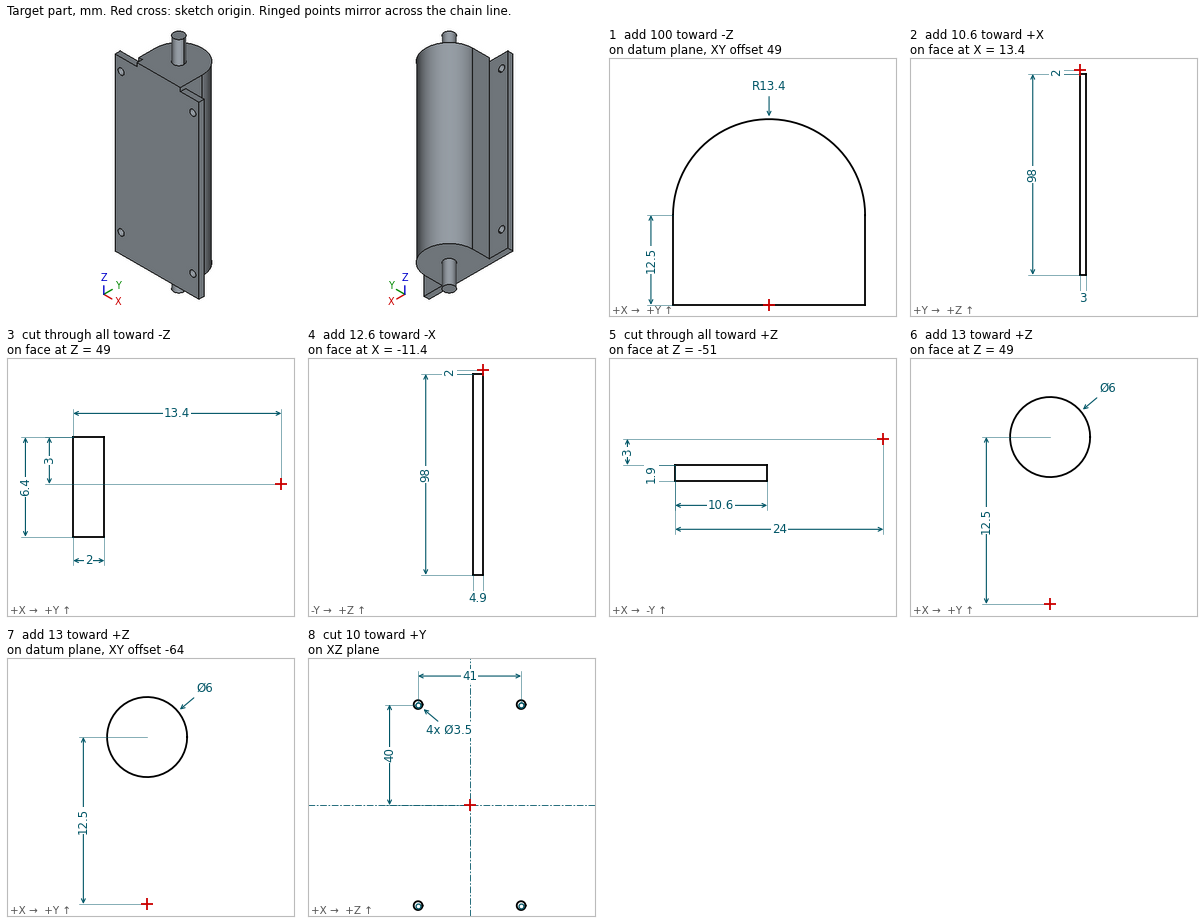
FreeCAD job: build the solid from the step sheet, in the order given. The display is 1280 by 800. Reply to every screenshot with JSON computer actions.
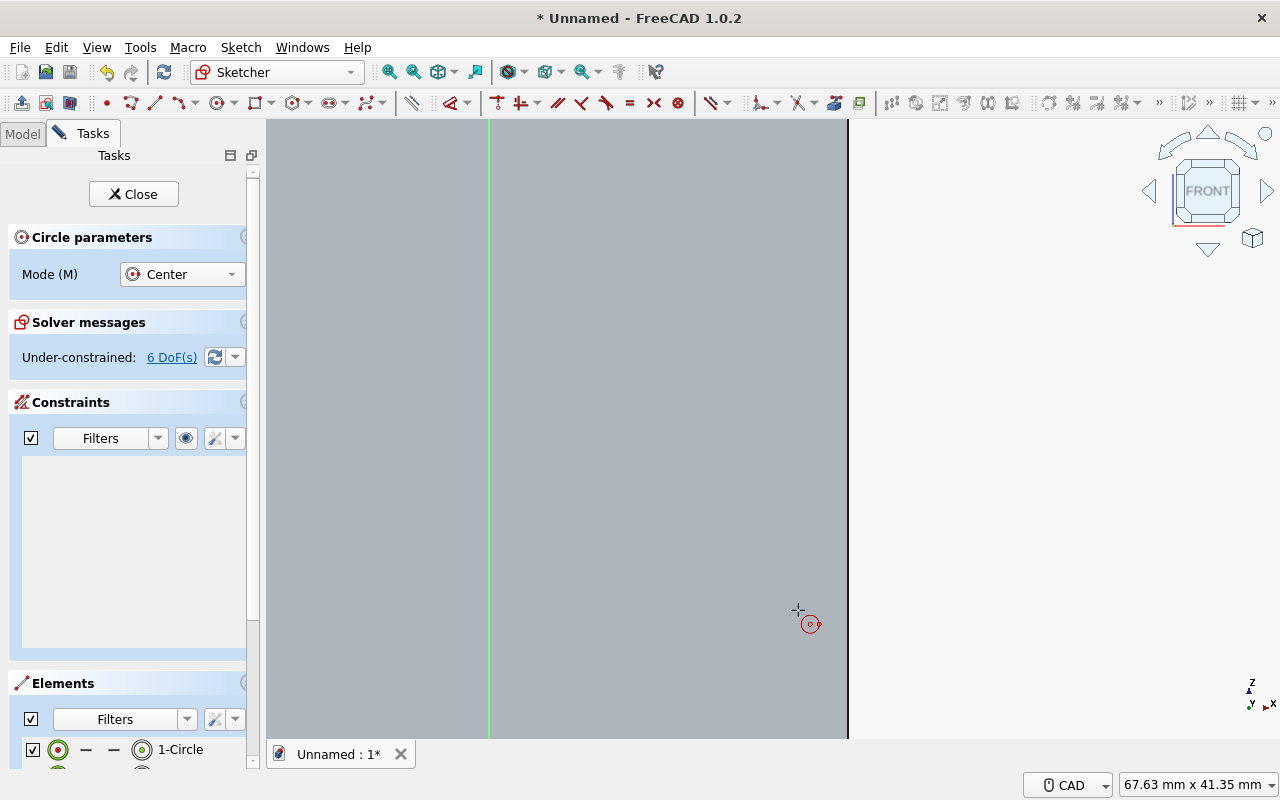
{"action": "left_click", "coordinate": [796, 608]}
{"action": "left_click", "coordinate": [814, 590]}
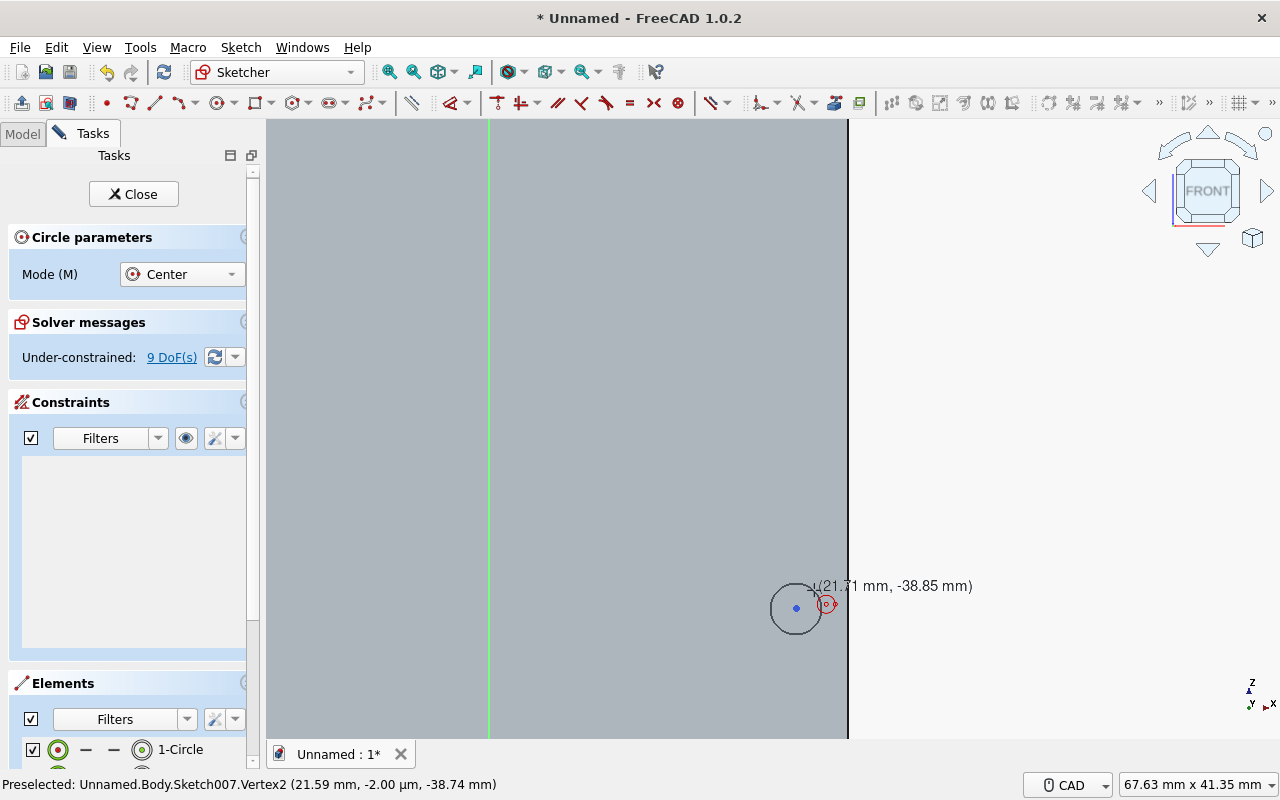
{"action": "scroll", "coordinate": [798, 610], "scroll_direction": "down", "scroll_amount": 6}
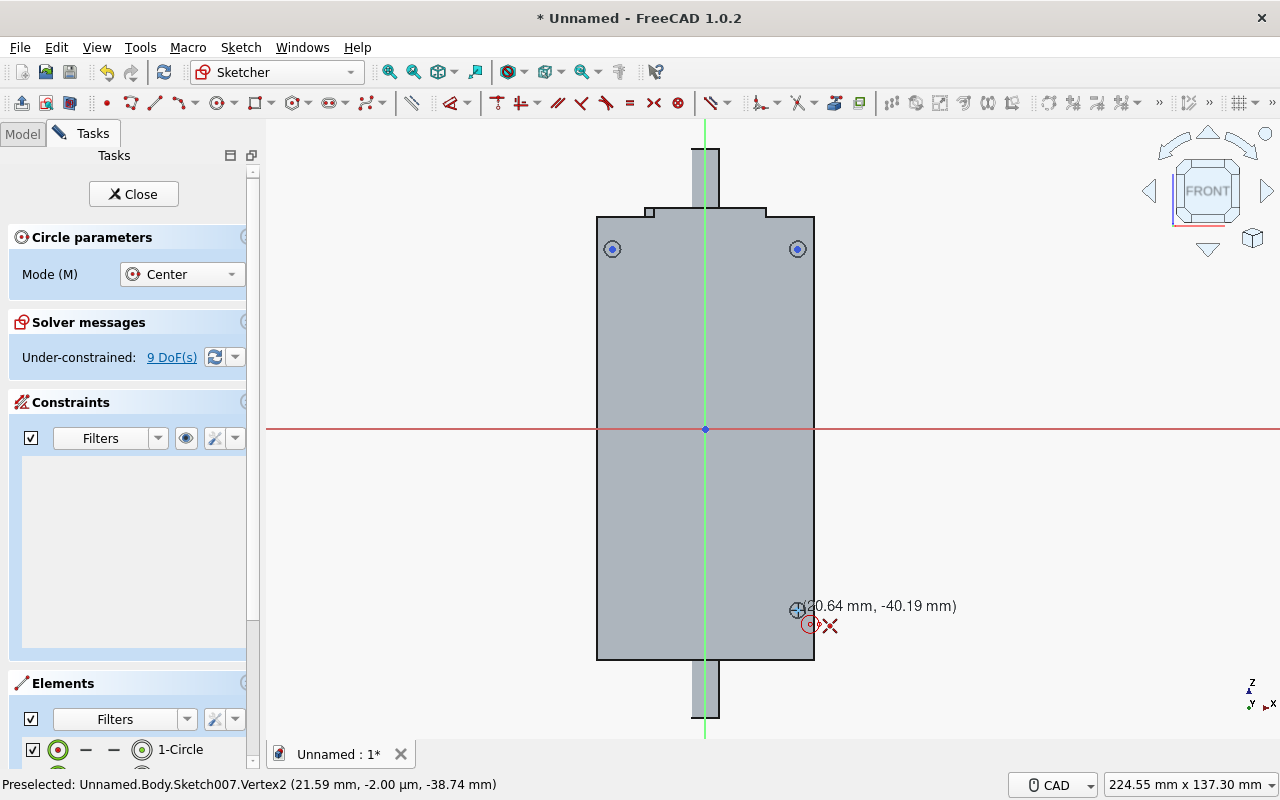
{"action": "scroll", "coordinate": [613, 610], "scroll_direction": "up", "scroll_amount": 6}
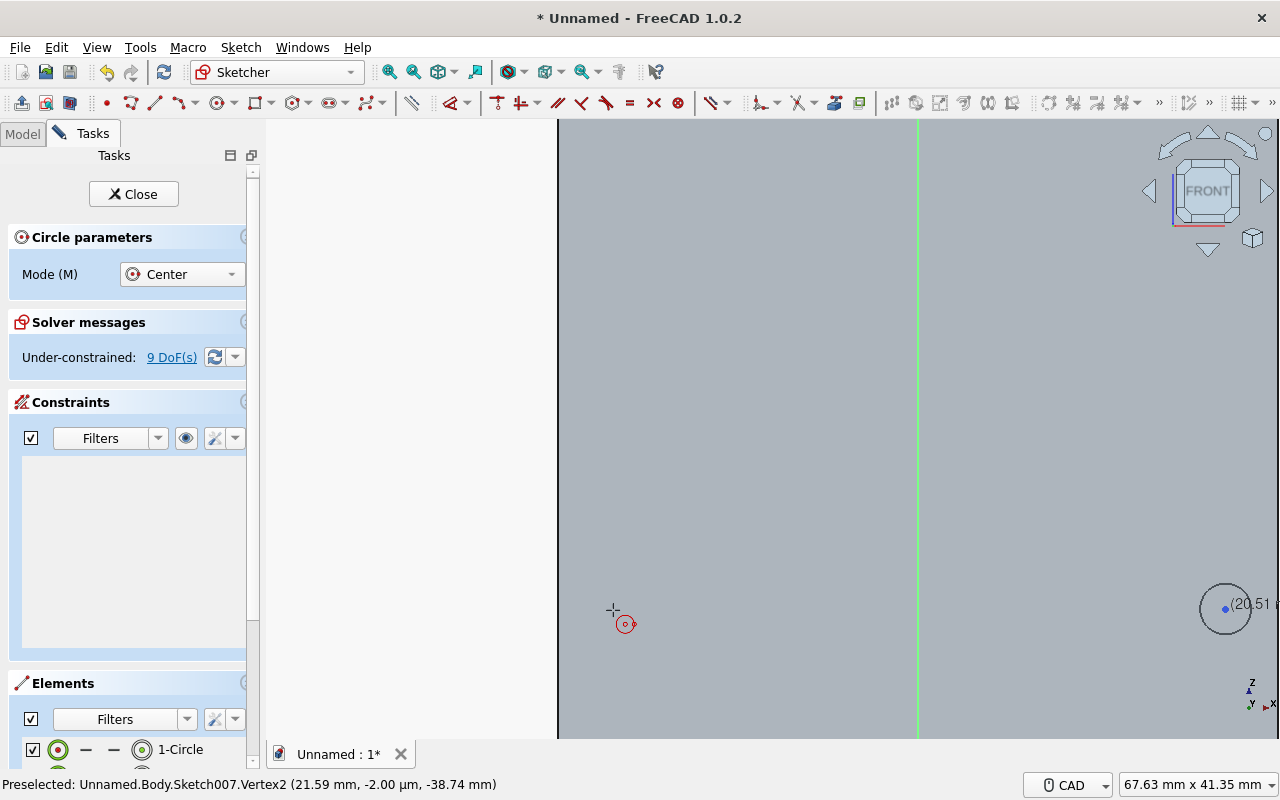
{"action": "left_click", "coordinate": [611, 608]}
{"action": "left_click", "coordinate": [629, 590]}
{"action": "key", "text": "Escape"}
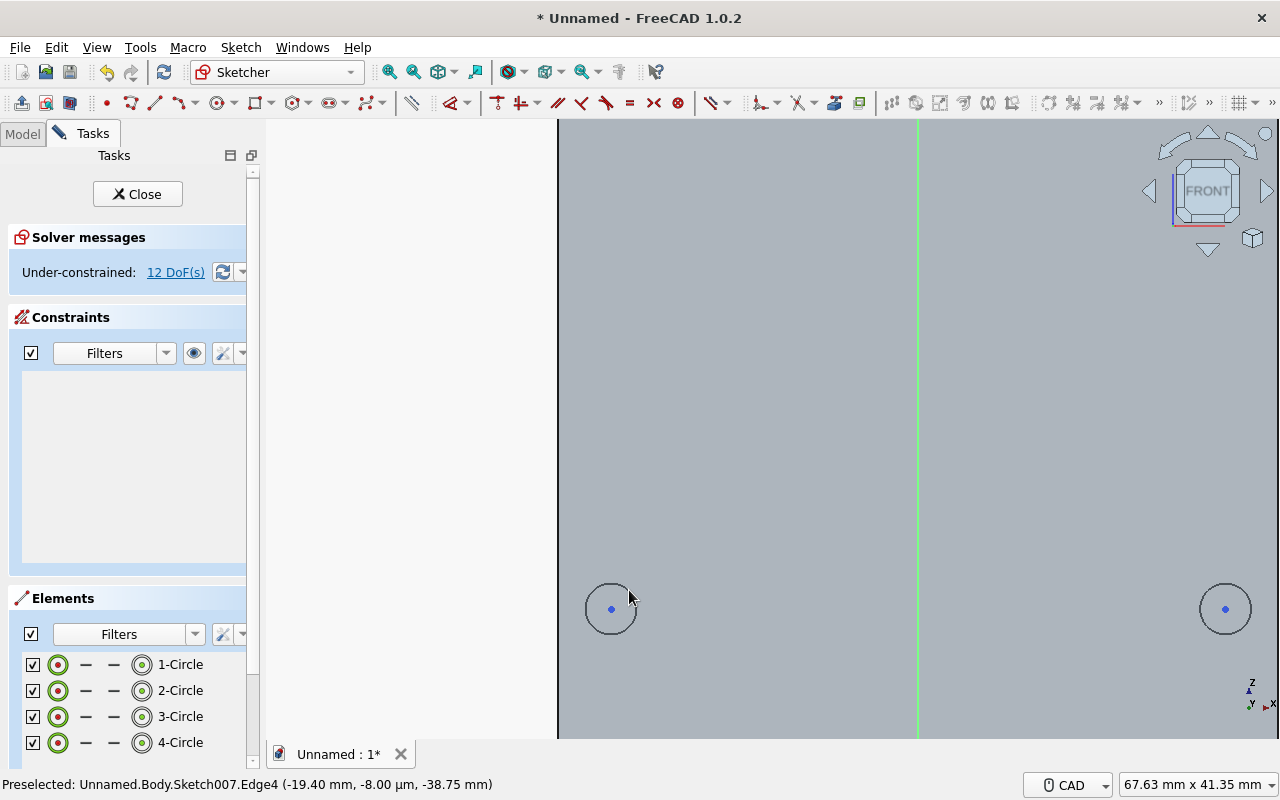
{"action": "scroll", "coordinate": [612, 610], "scroll_direction": "down", "scroll_amount": 6}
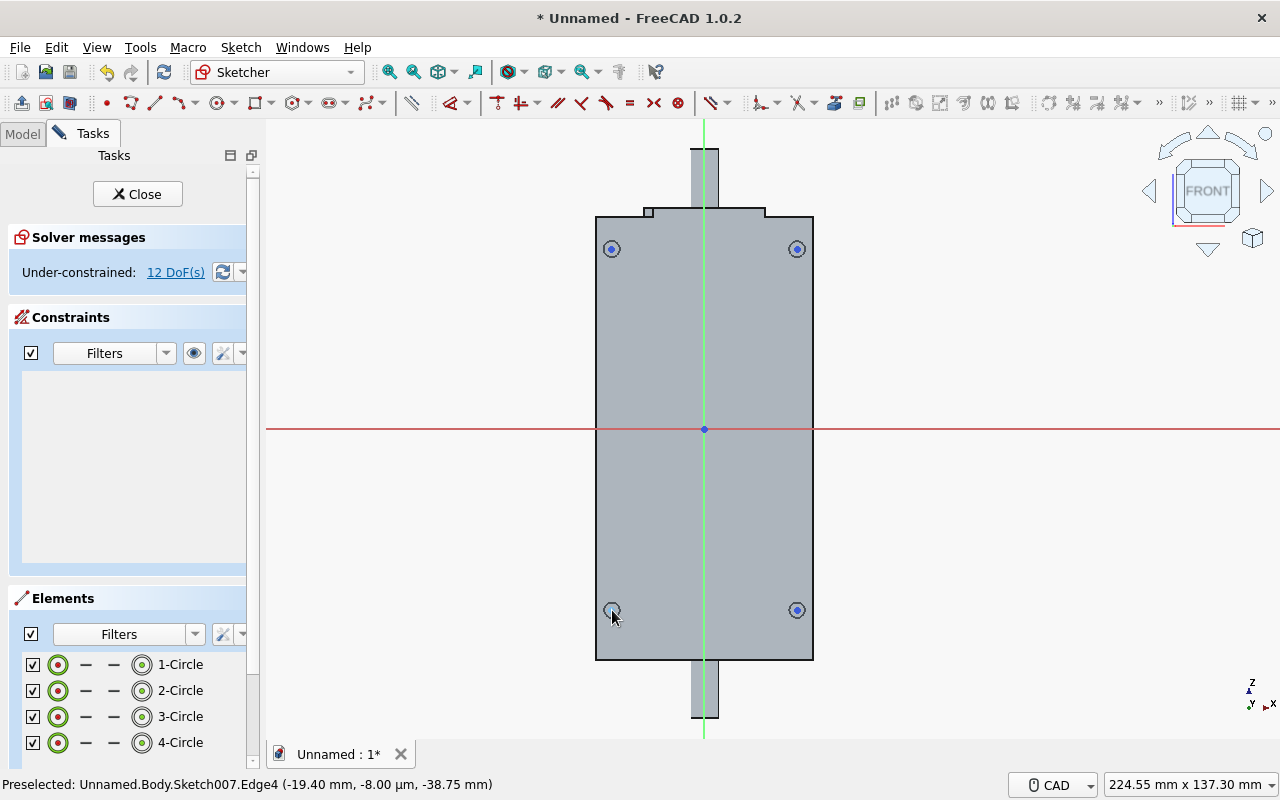
{"action": "scroll", "coordinate": [617, 243], "scroll_direction": "up", "scroll_amount": 3}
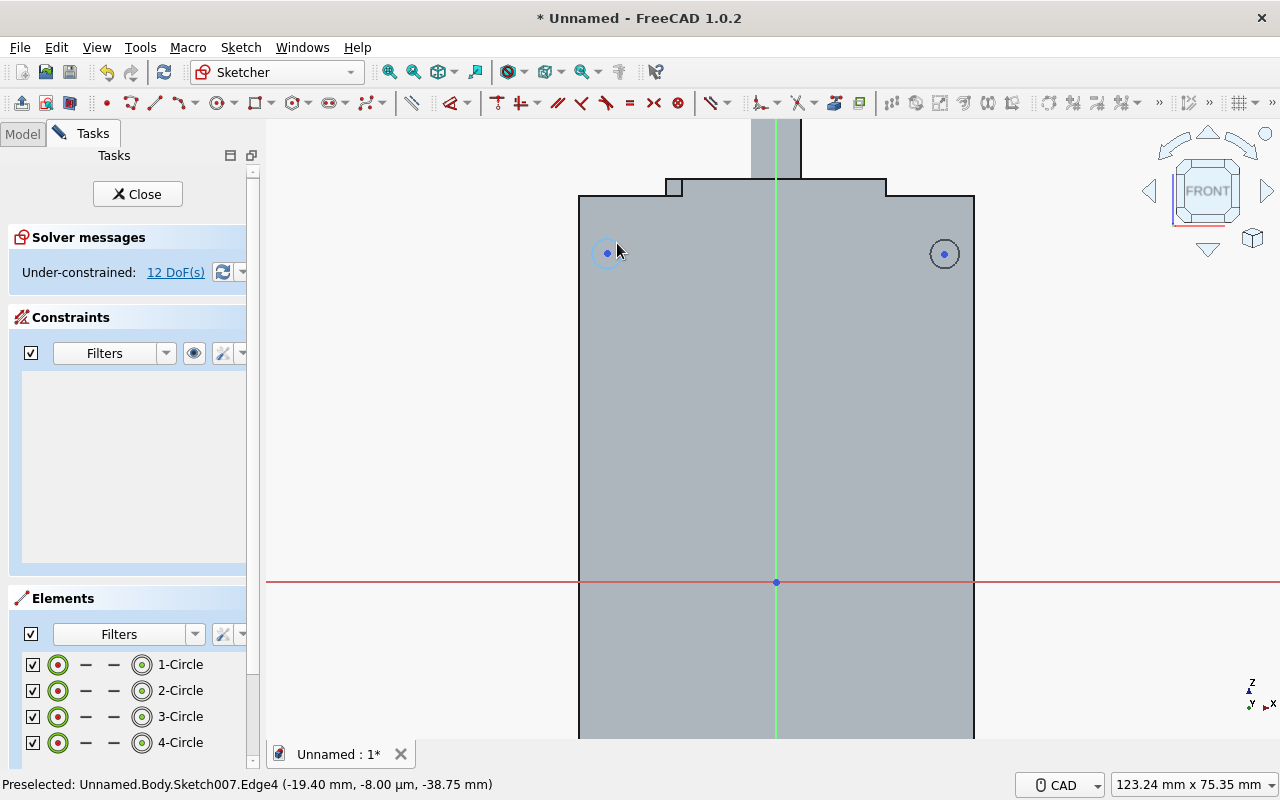
{"action": "left_click", "coordinate": [618, 243]}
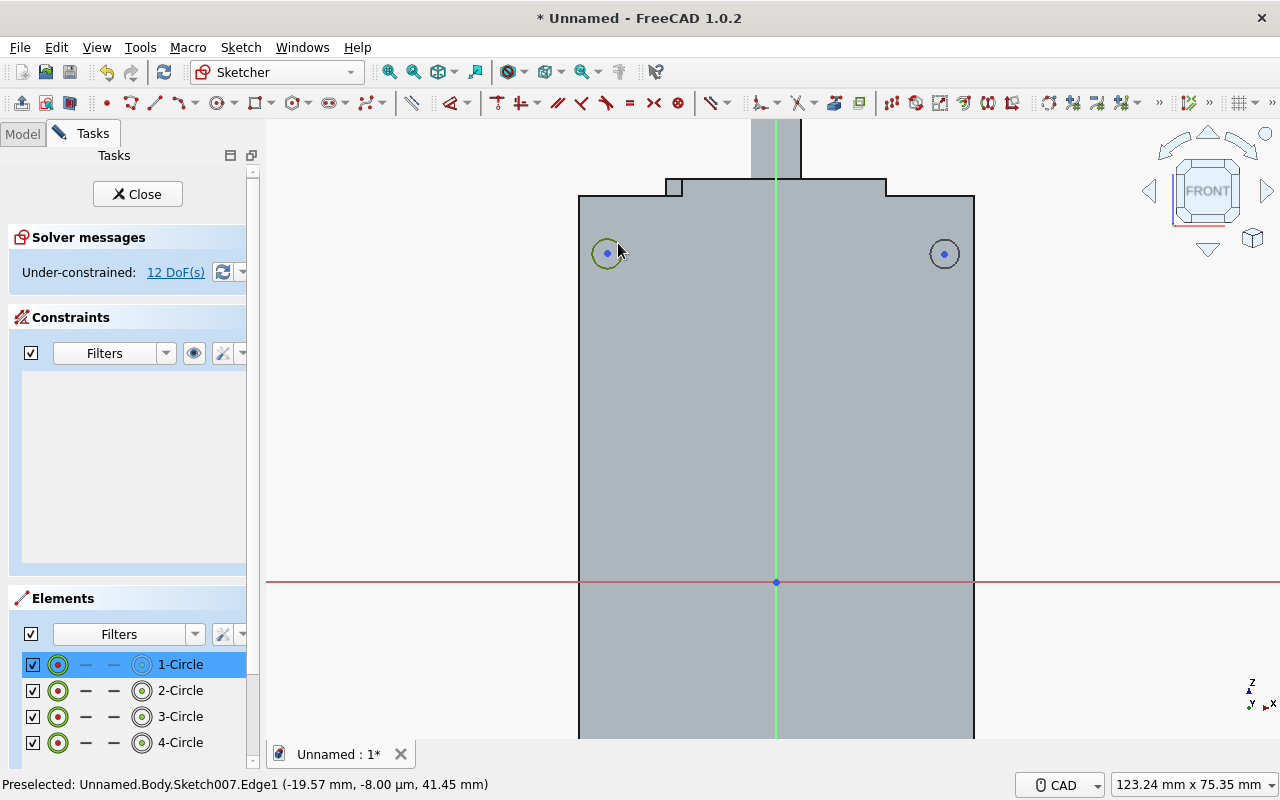
{"action": "left_click", "coordinate": [955, 244]}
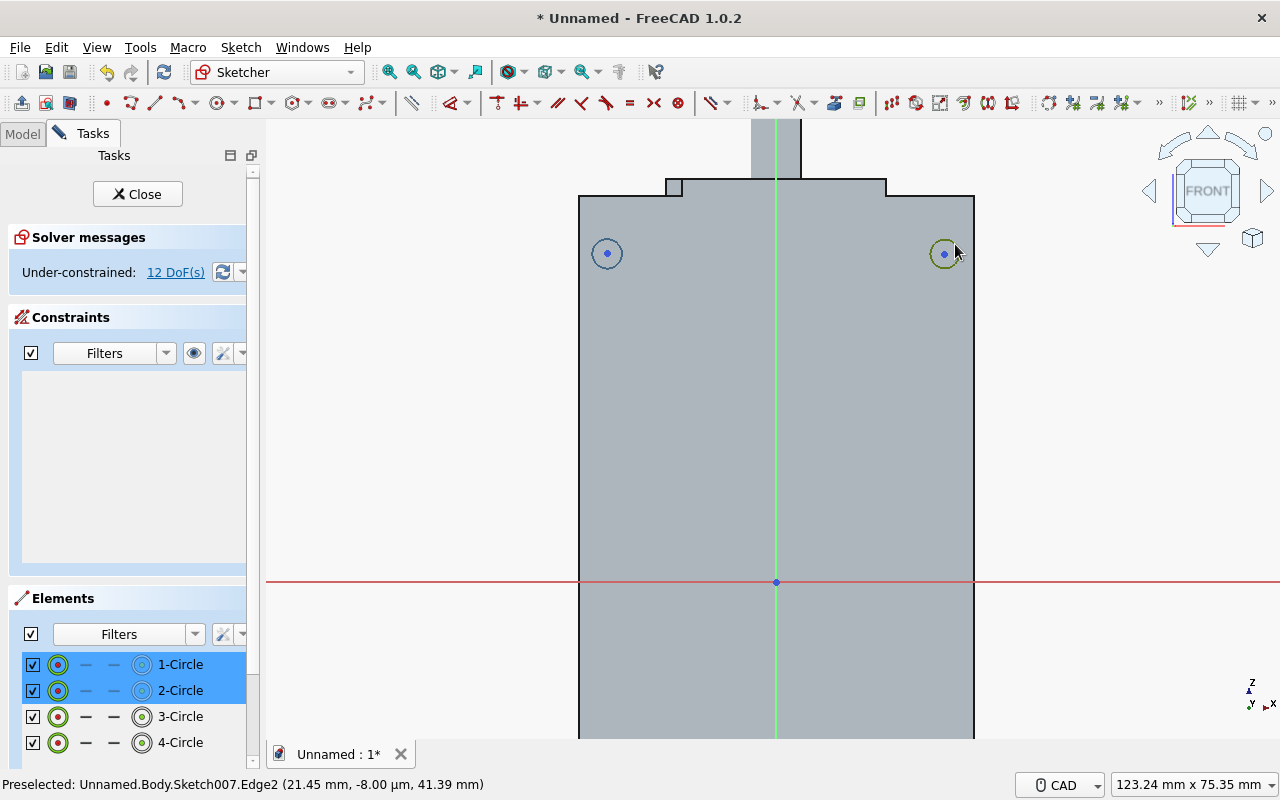
{"action": "scroll", "coordinate": [617, 242], "scroll_direction": "down", "scroll_amount": 3}